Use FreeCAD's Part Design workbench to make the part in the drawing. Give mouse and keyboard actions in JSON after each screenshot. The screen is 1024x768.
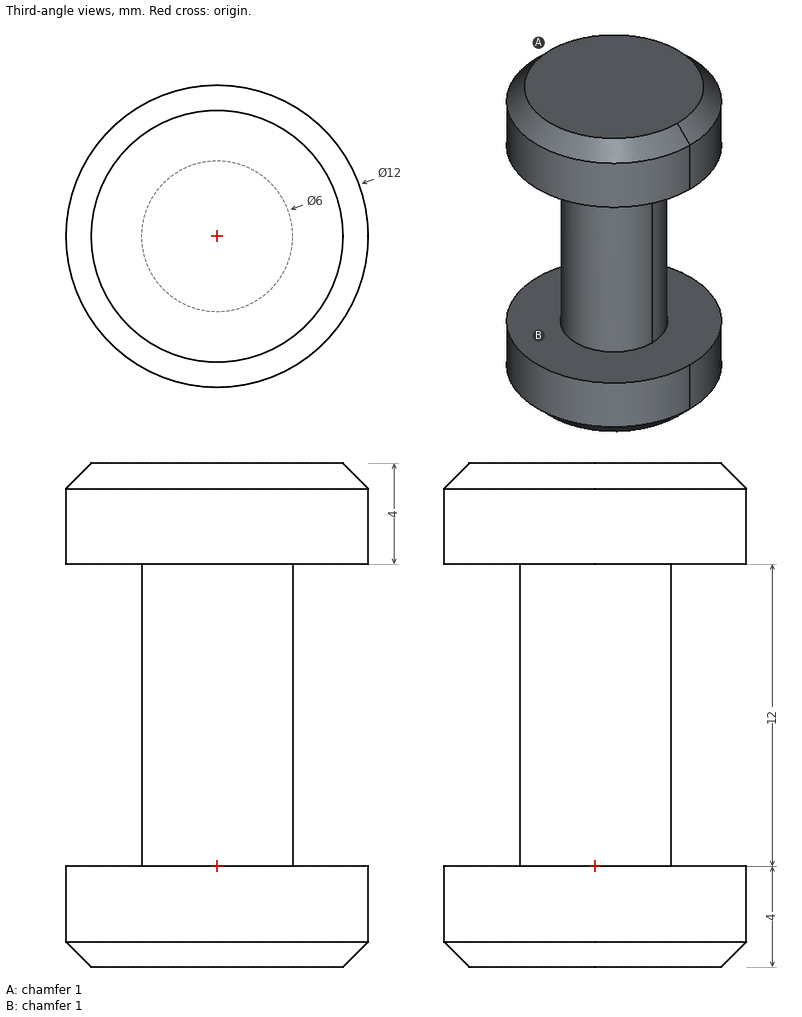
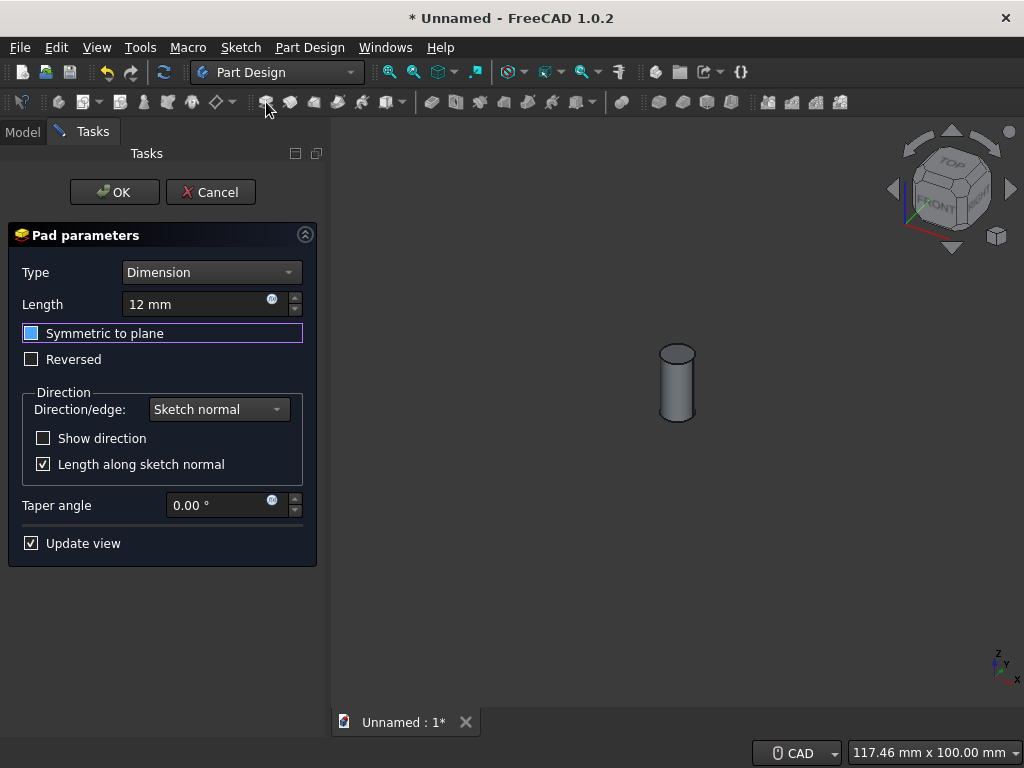
{"action": "left_click", "coordinate": [115, 192]}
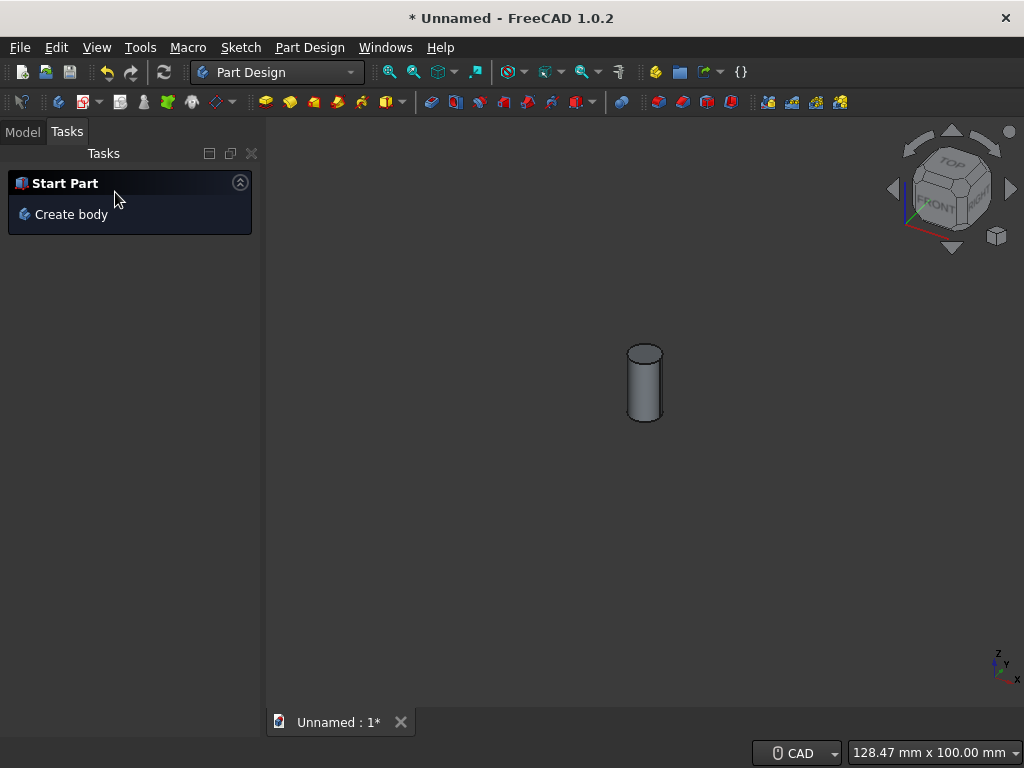
{"action": "key", "text": "v f"}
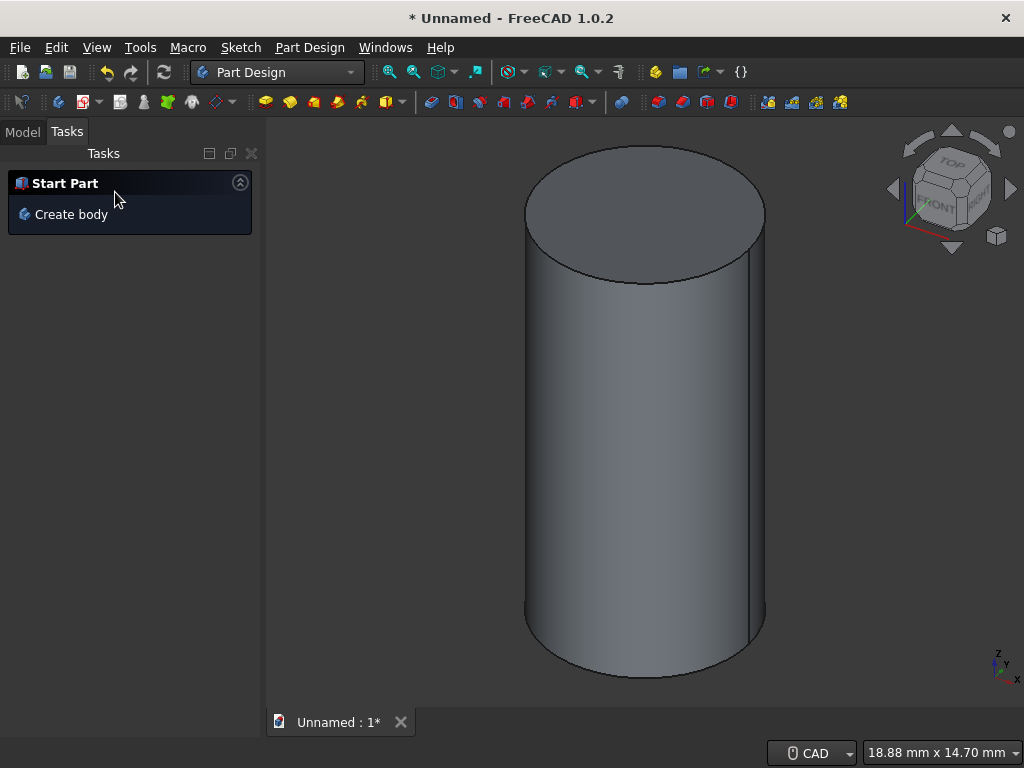
{"action": "left_click", "coordinate": [645, 214]}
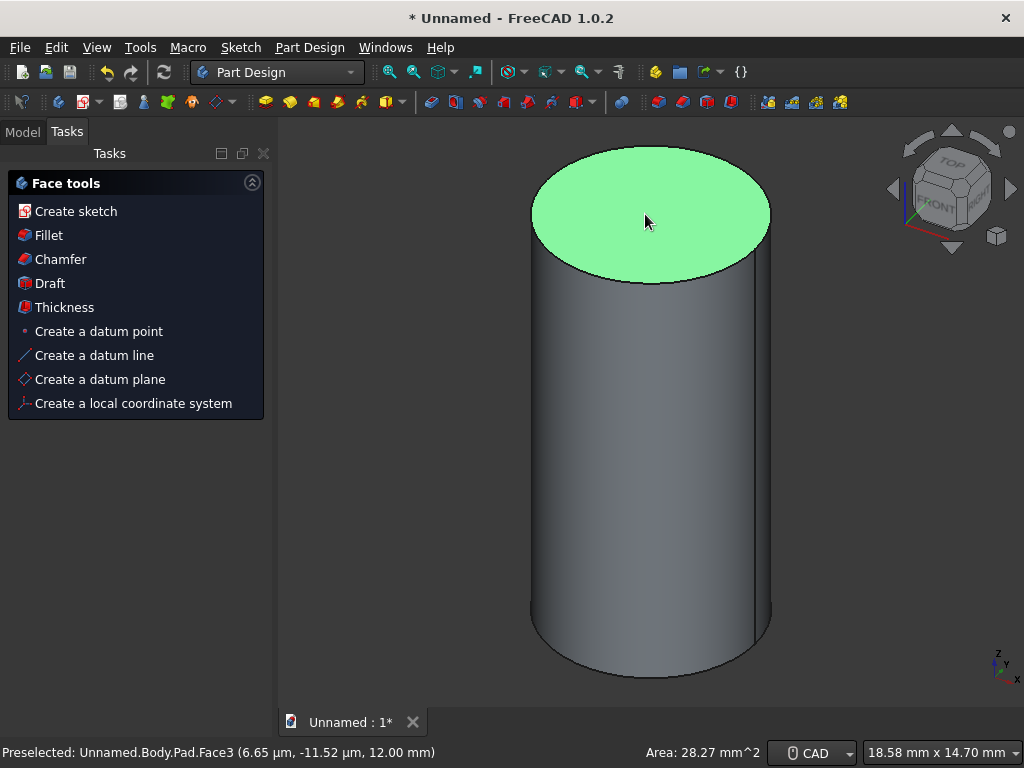
{"action": "left_click", "coordinate": [84, 102]}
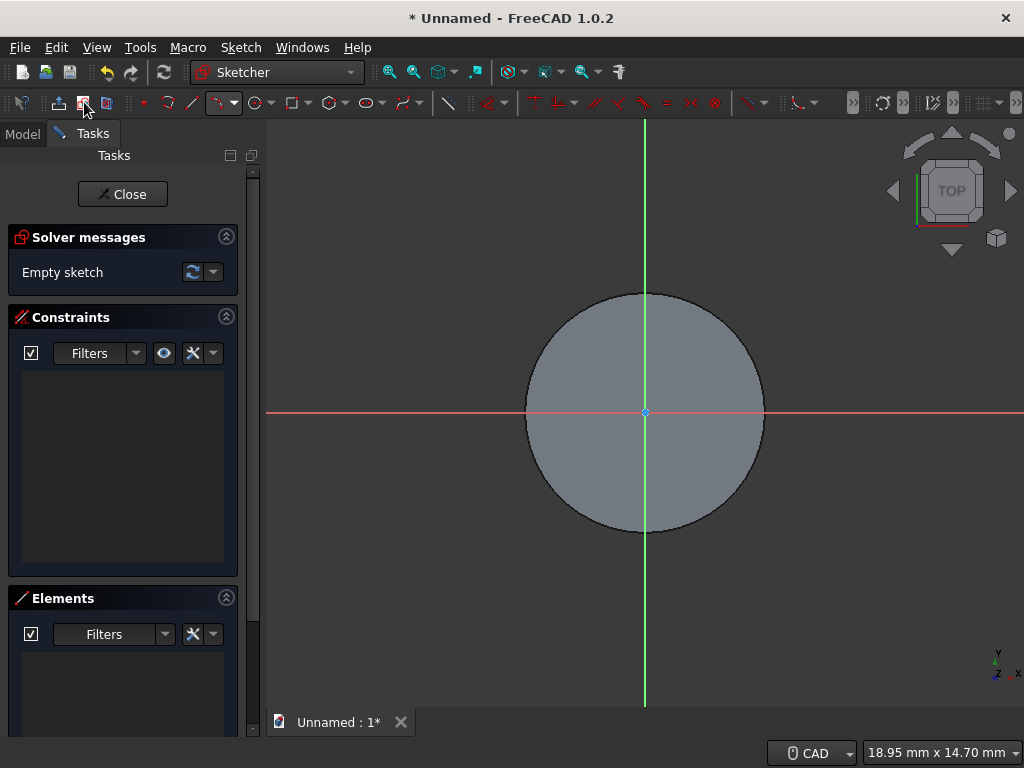
{"action": "scroll", "coordinate": [294, 413], "scroll_direction": "down", "scroll_amount": 1}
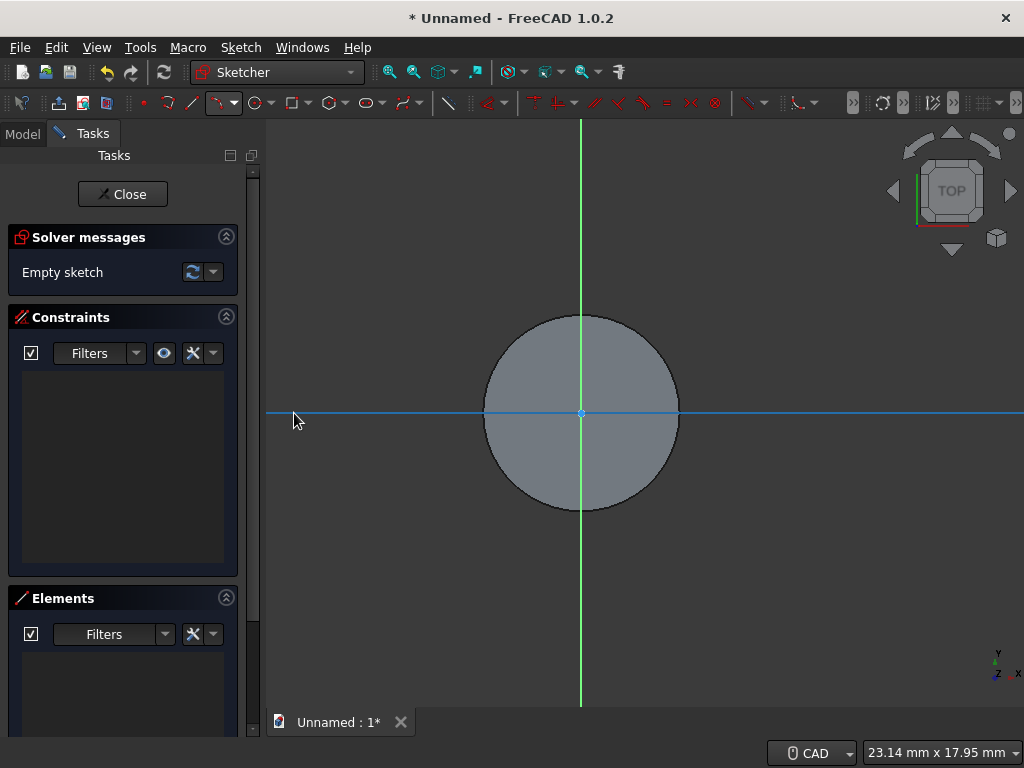
{"action": "left_click", "coordinate": [256, 104]}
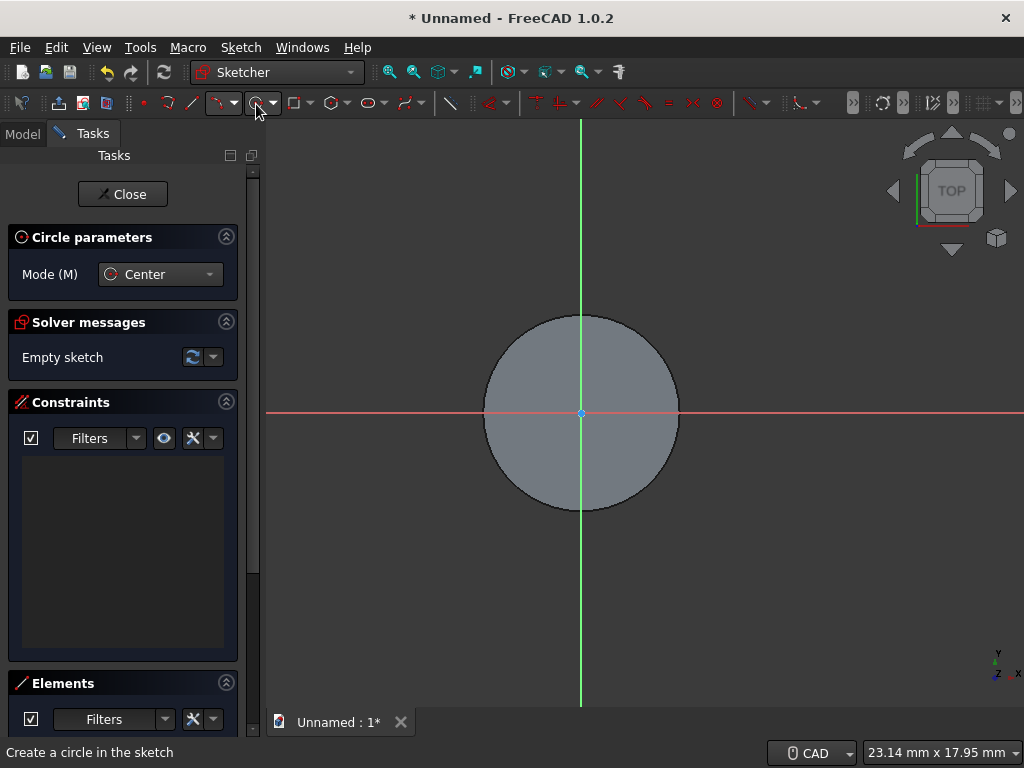
{"action": "left_click", "coordinate": [581, 413]}
{"action": "left_click", "coordinate": [720, 274]}
{"action": "key", "text": "Escape"}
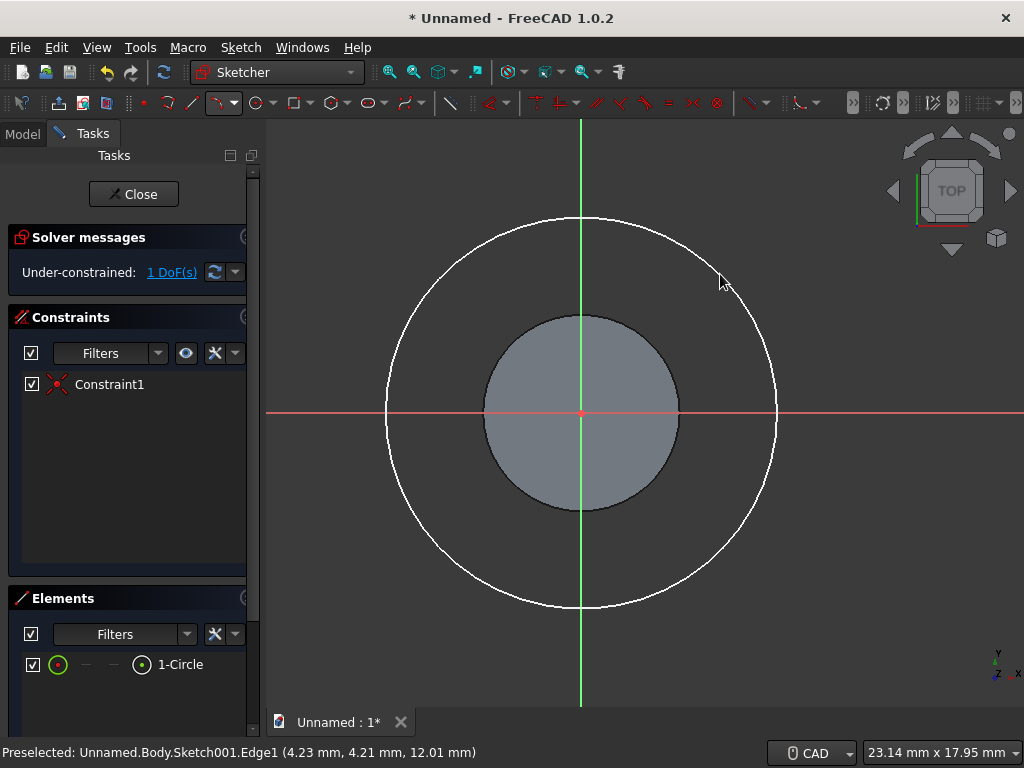
{"action": "key", "text": "d"}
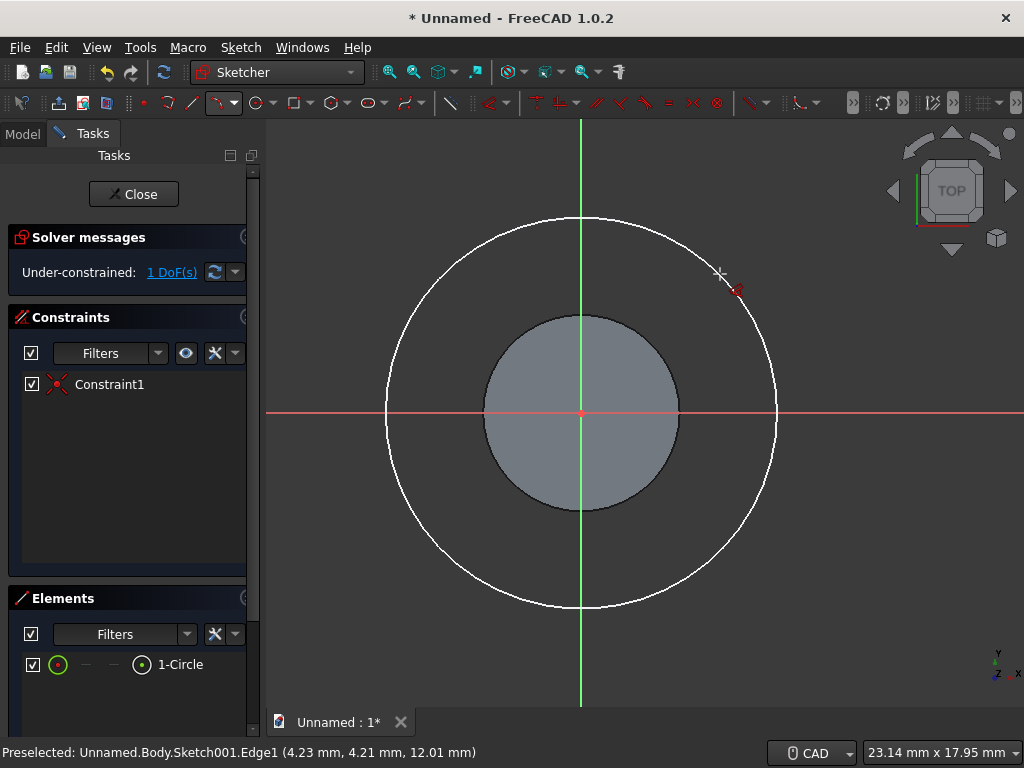
{"action": "left_click", "coordinate": [719, 274]}
{"action": "left_click", "coordinate": [742, 251]}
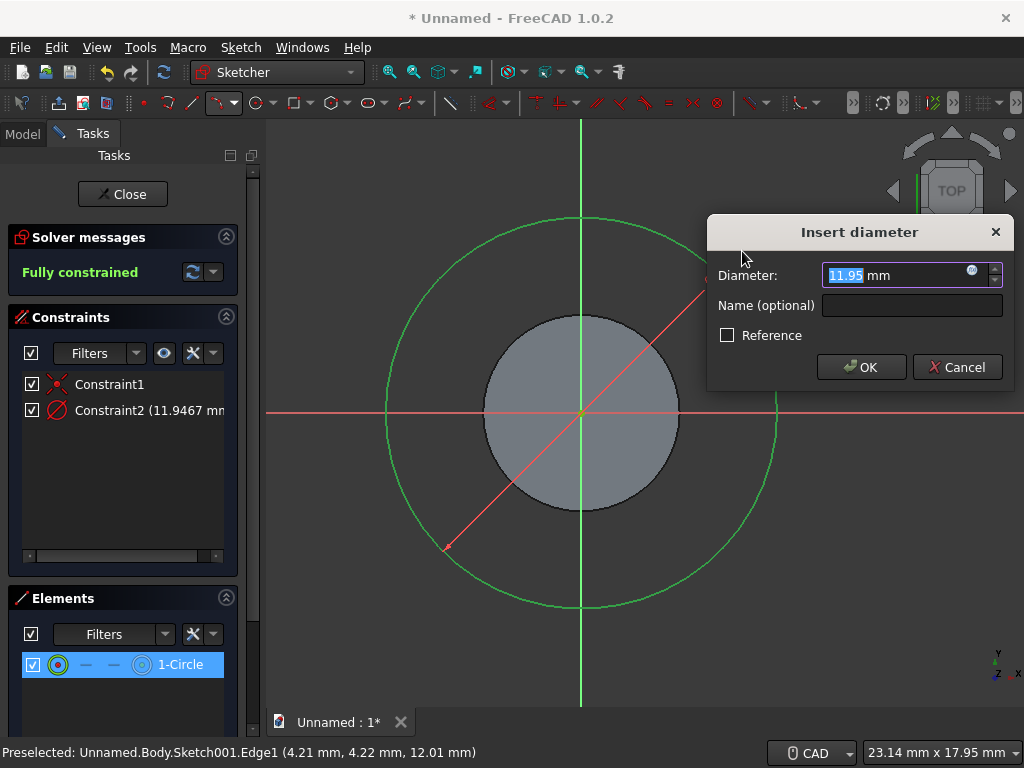
{"action": "type", "text": "12"}
{"action": "key", "text": "Return"}
{"action": "key", "text": "Escape"}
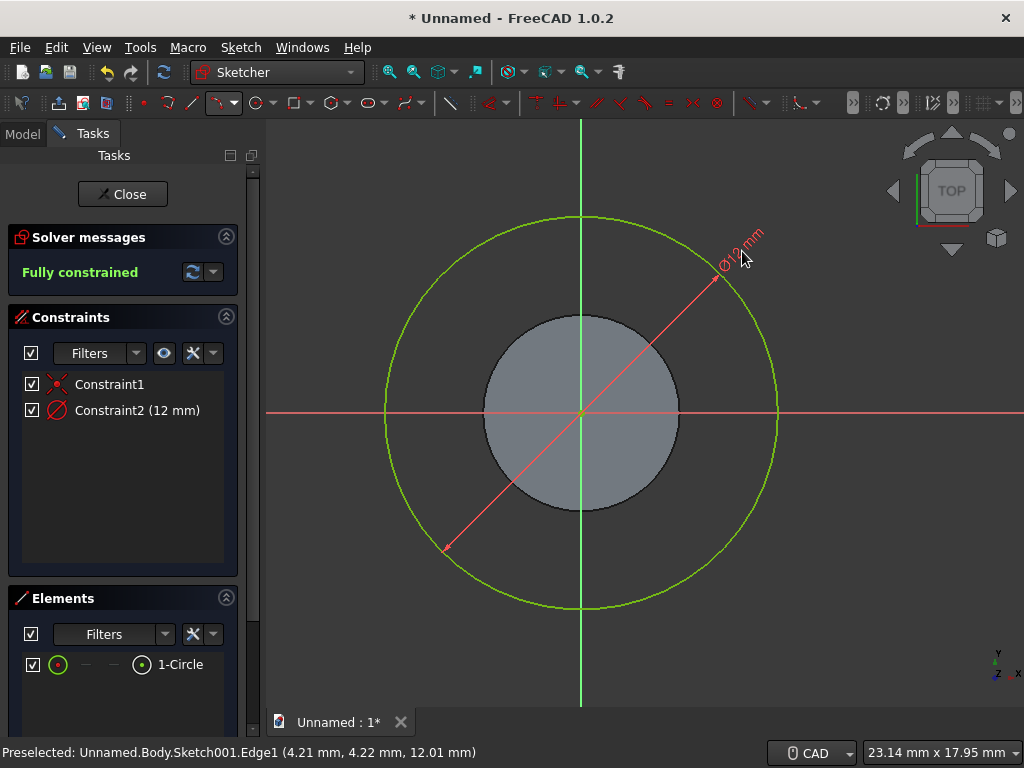
{"action": "left_click", "coordinate": [123, 194]}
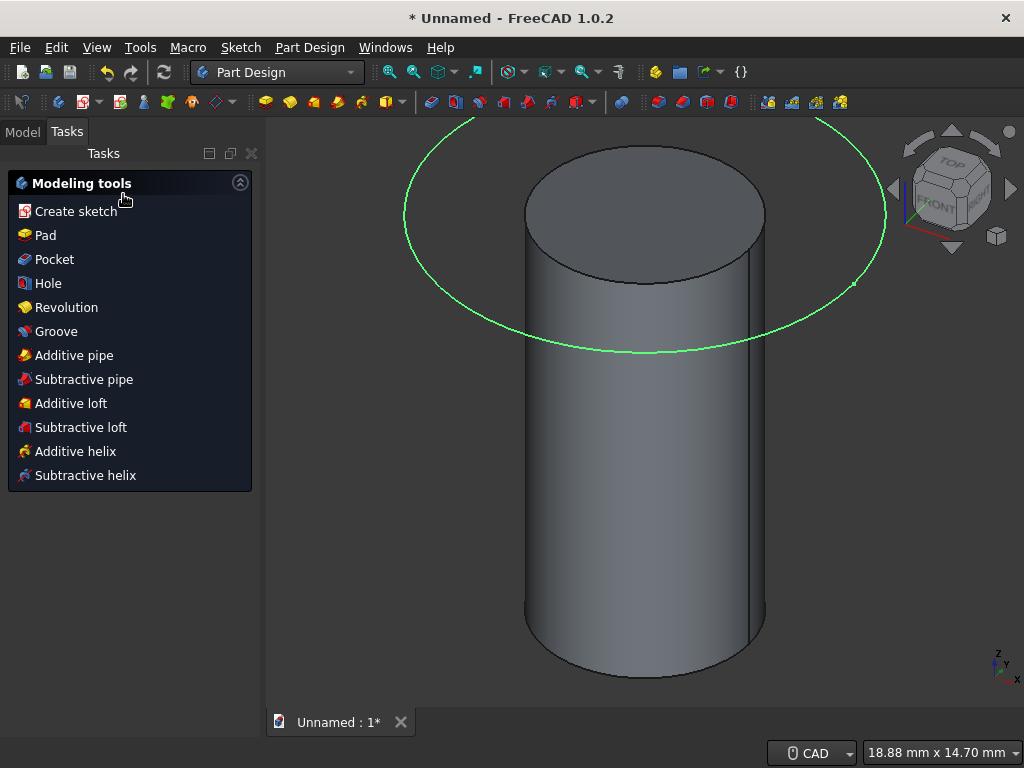
{"action": "left_click", "coordinate": [266, 102]}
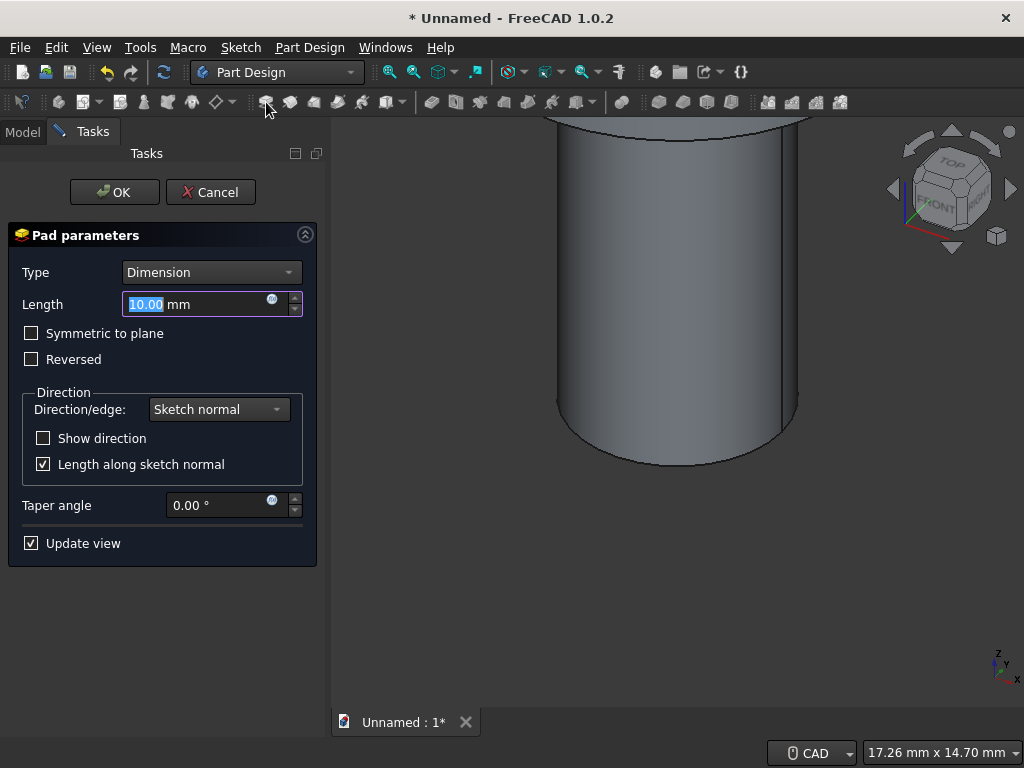
{"action": "type", "text": "4"}
{"action": "key", "text": "Tab"}